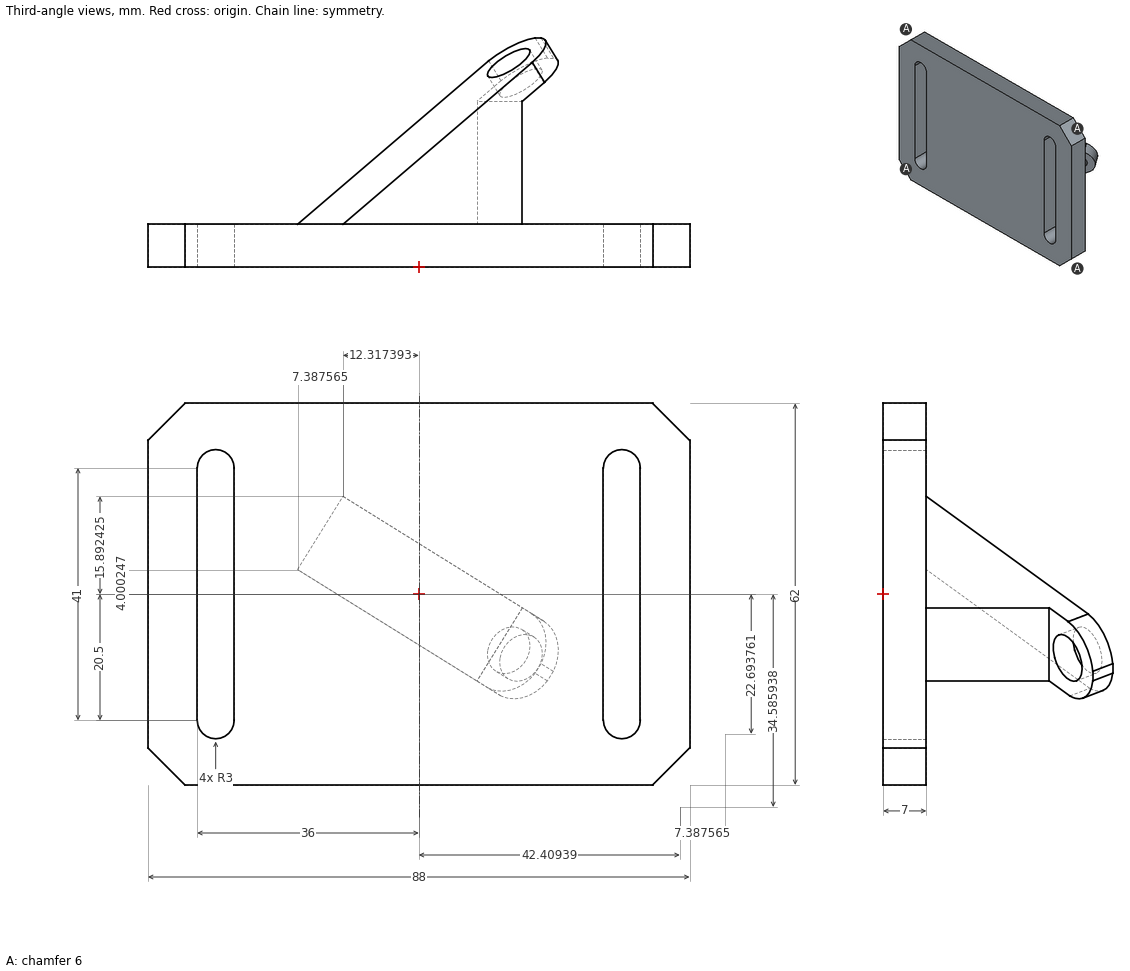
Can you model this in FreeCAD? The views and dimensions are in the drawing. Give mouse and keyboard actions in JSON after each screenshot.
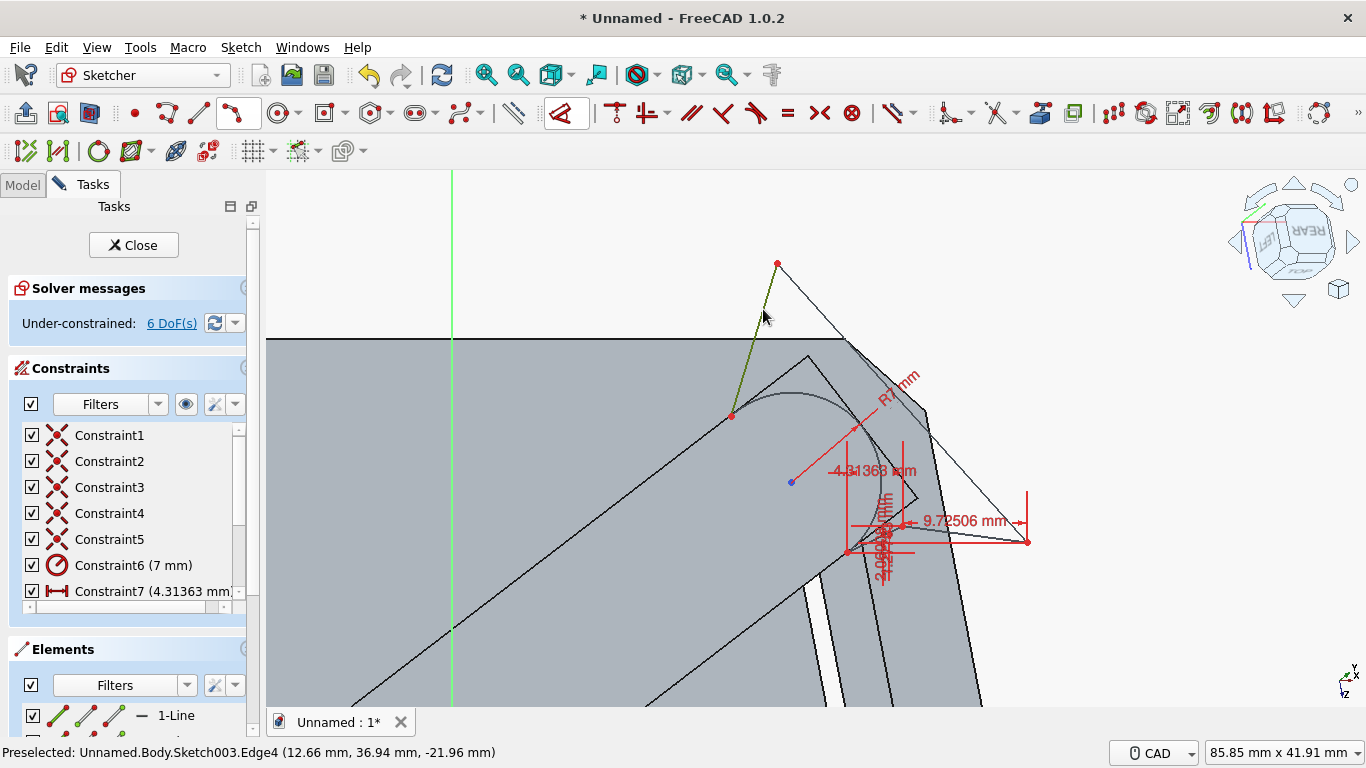
{"action": "key", "text": "l"}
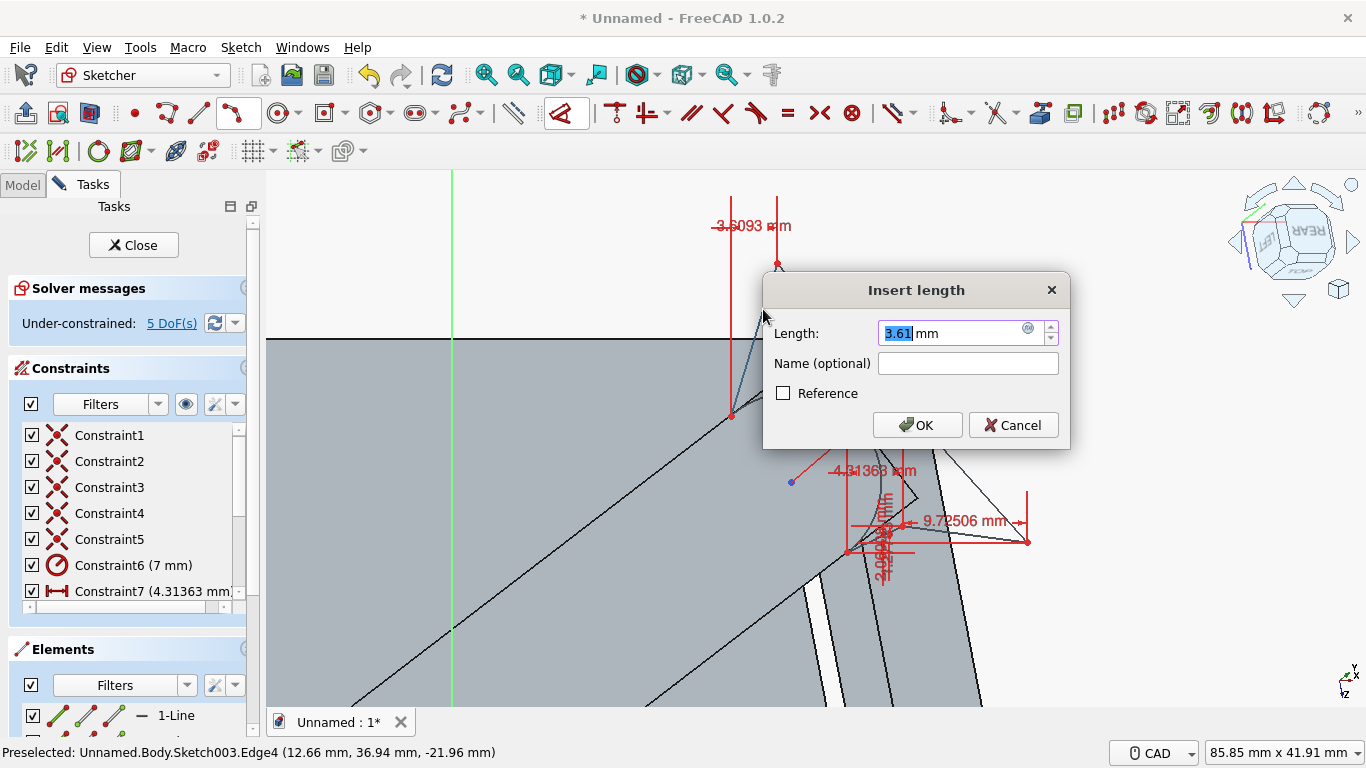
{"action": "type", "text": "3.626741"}
{"action": "key", "text": "Return"}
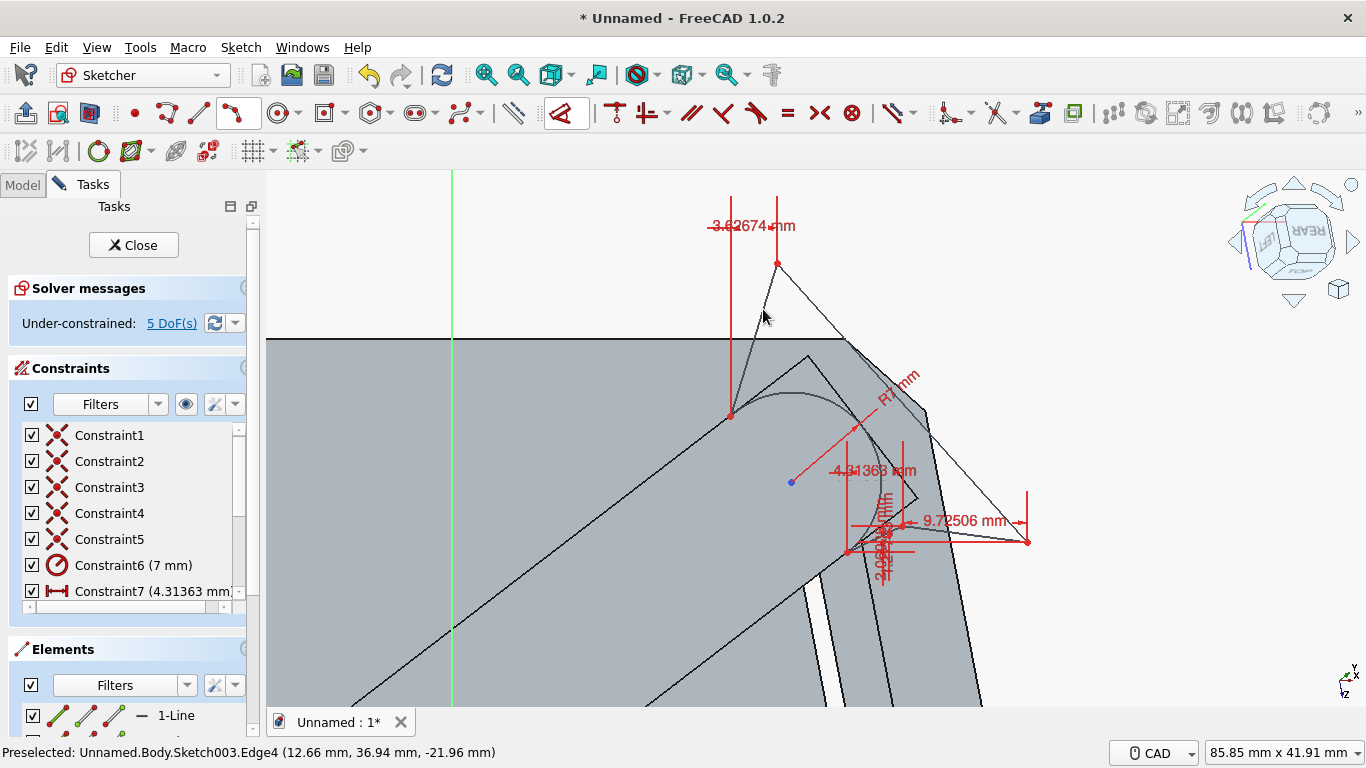
{"action": "left_click", "coordinate": [847, 552]}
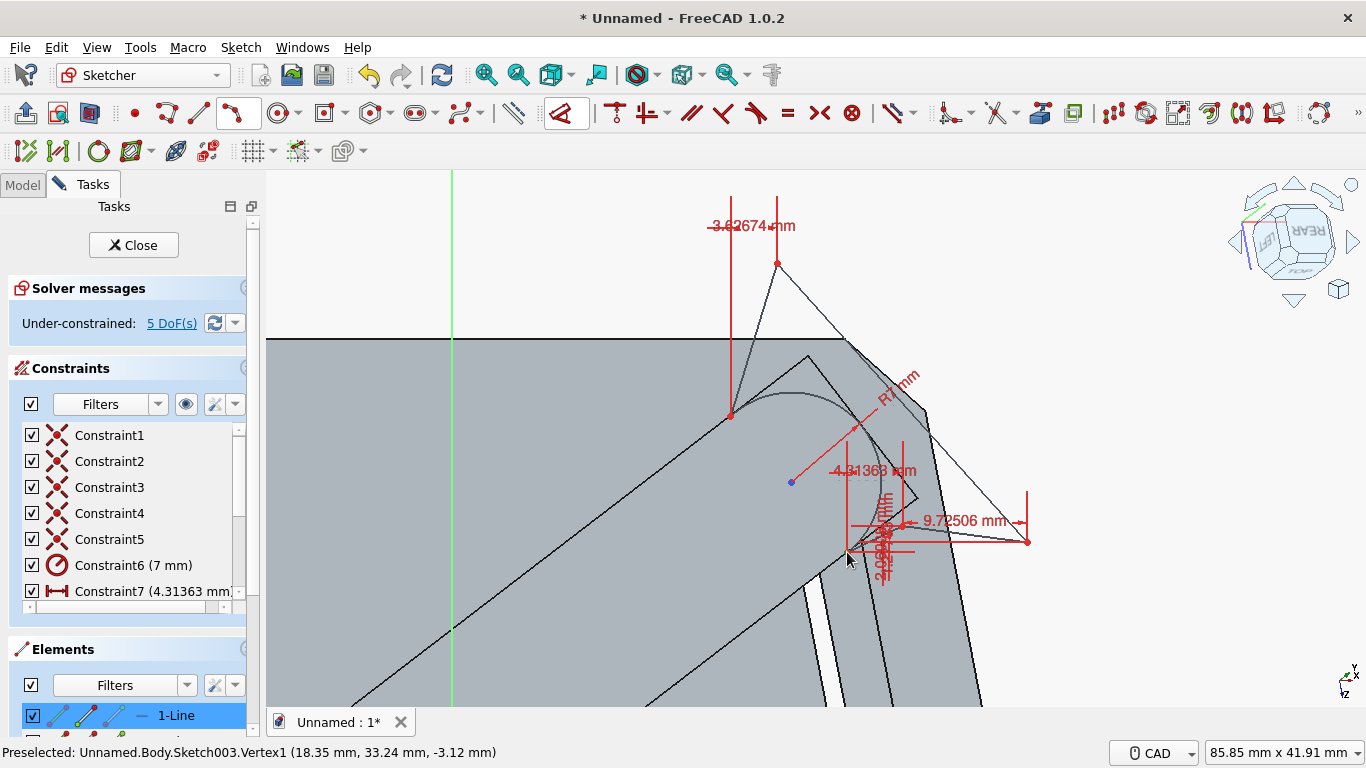
{"action": "key", "text": "l"}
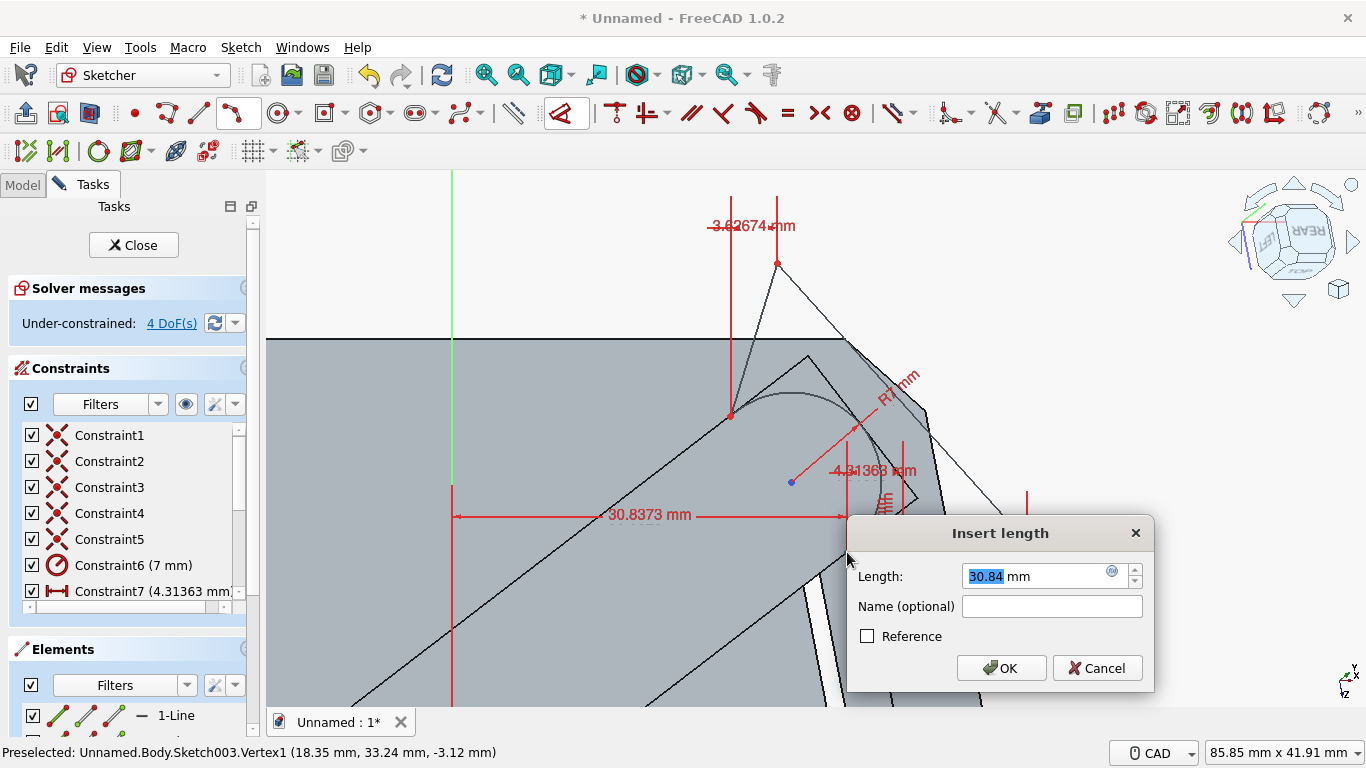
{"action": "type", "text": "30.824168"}
{"action": "key", "text": "Return"}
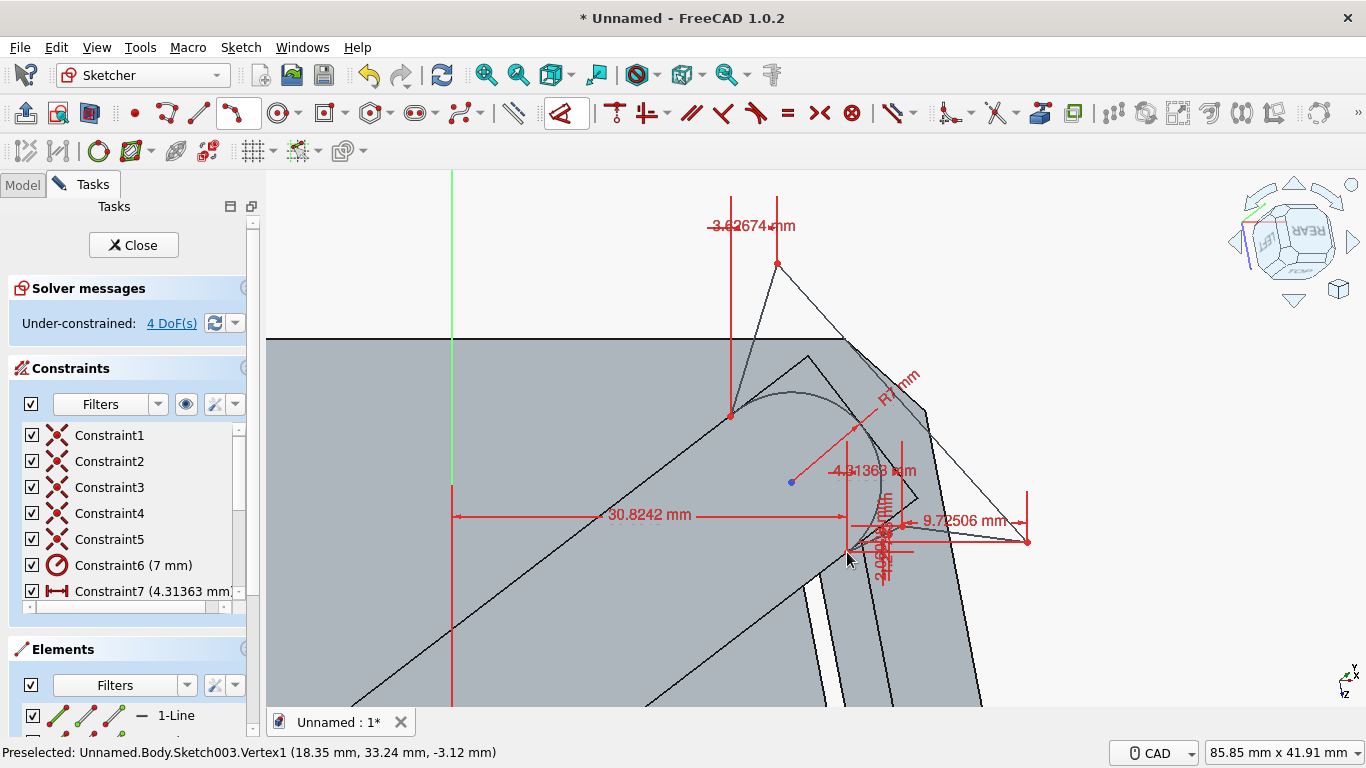
{"action": "left_click", "coordinate": [847, 552]}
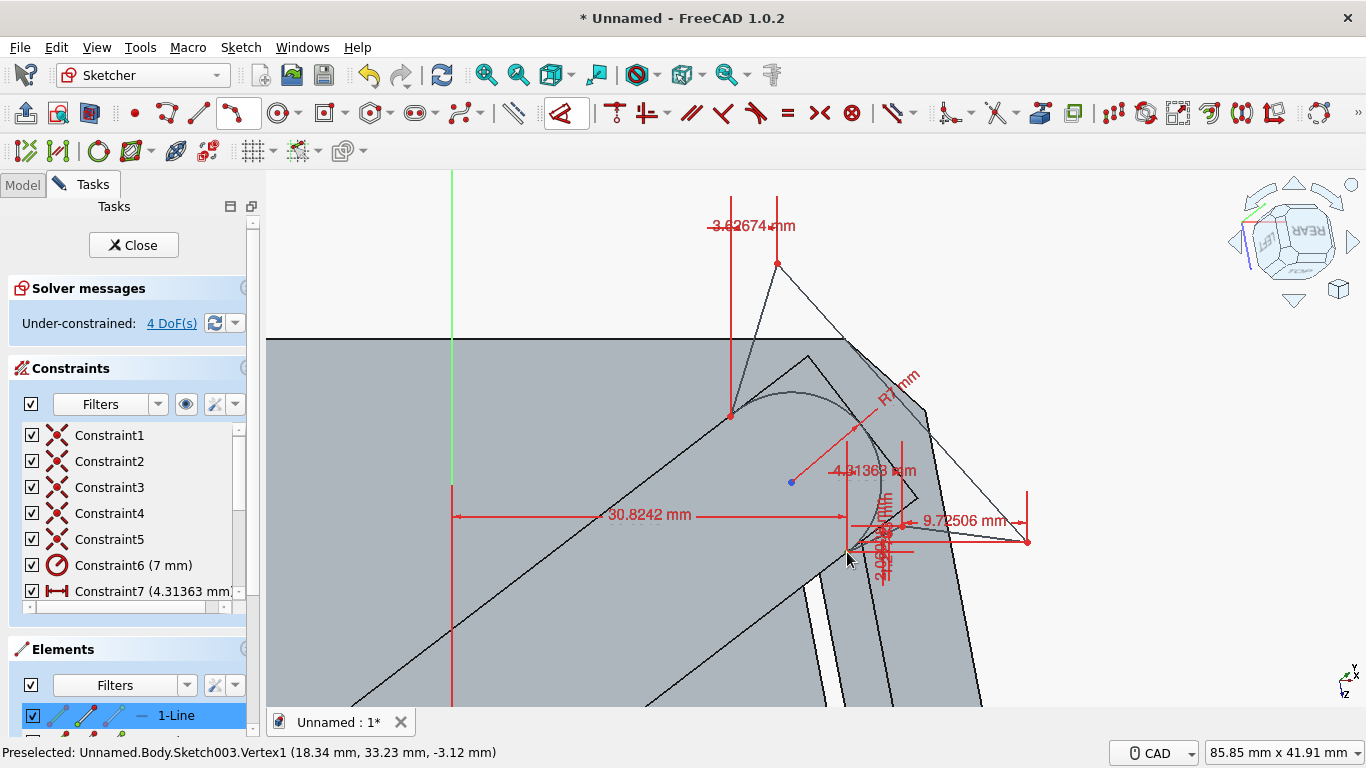
{"action": "left_click", "coordinate": [584, 114]}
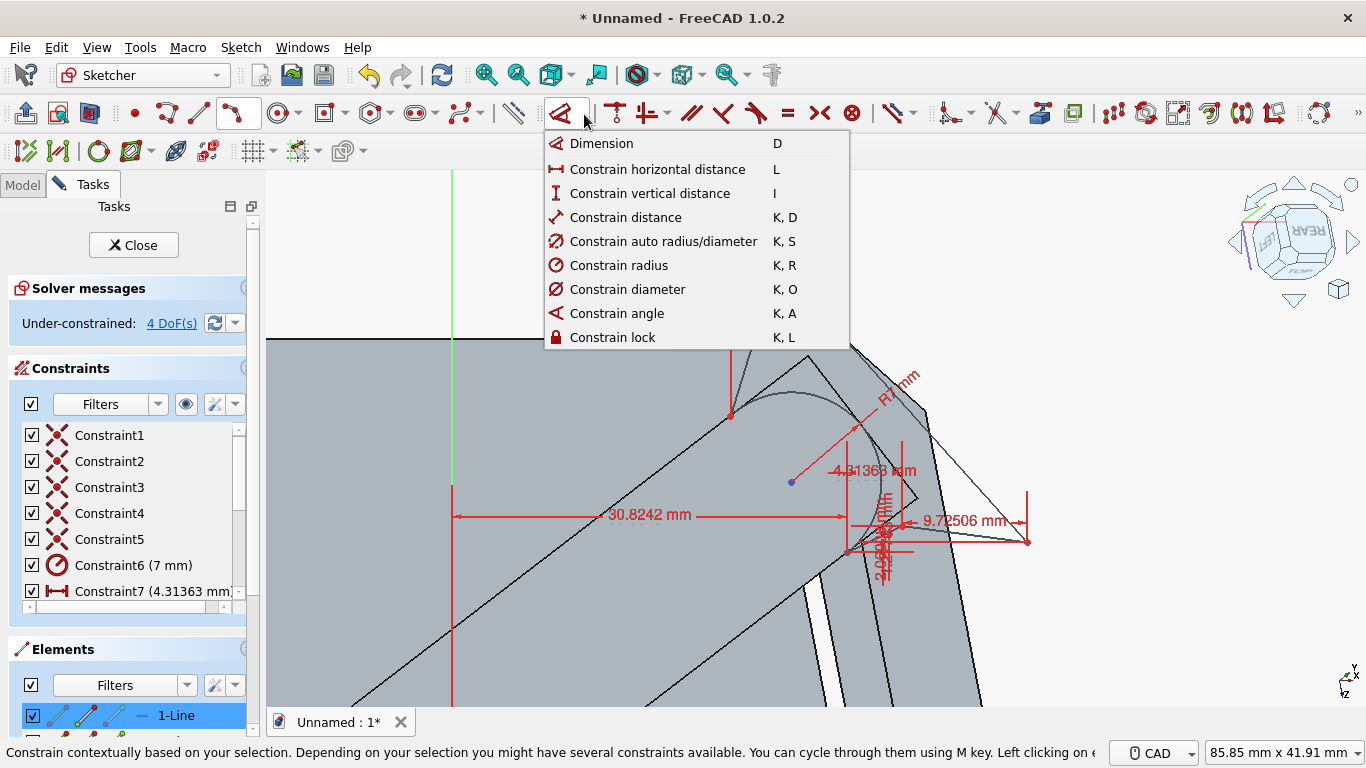
{"action": "left_click", "coordinate": [697, 193]}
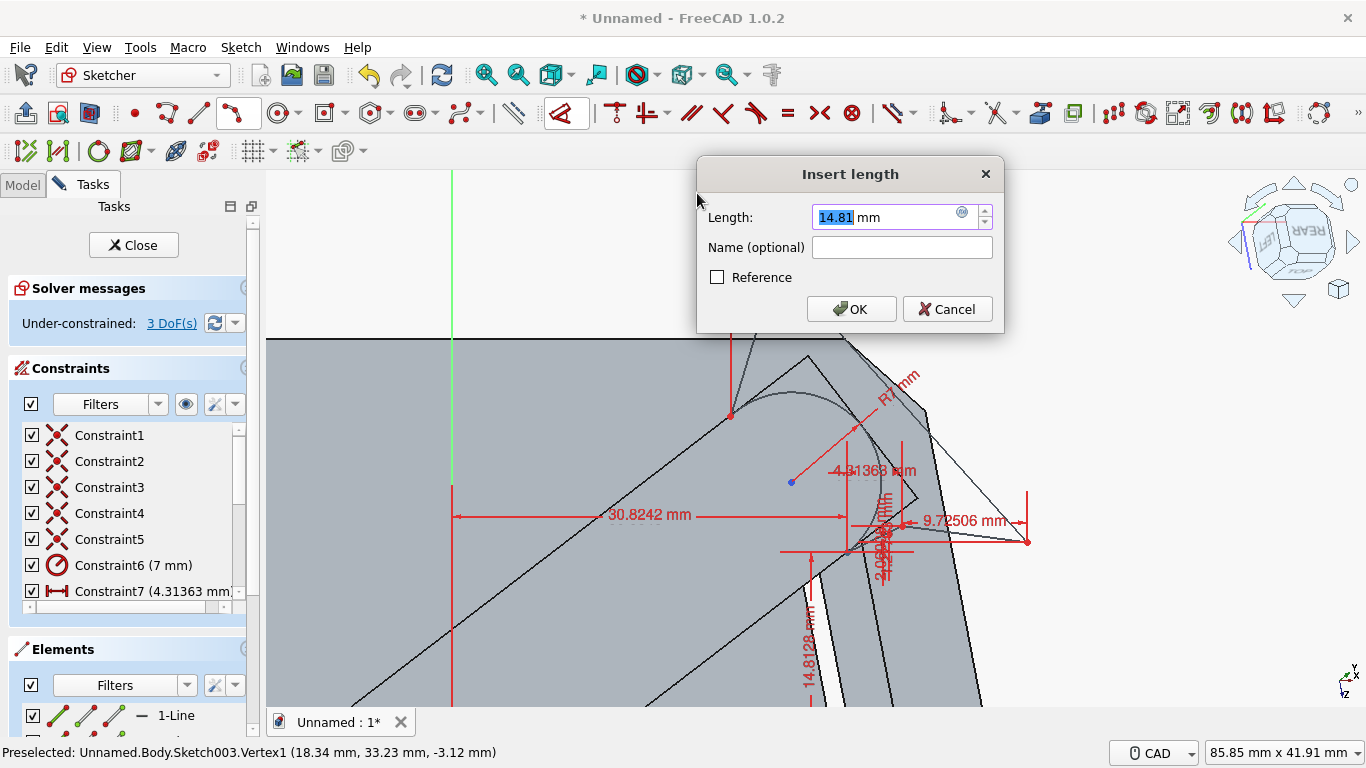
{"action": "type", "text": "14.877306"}
{"action": "key", "text": "Return"}